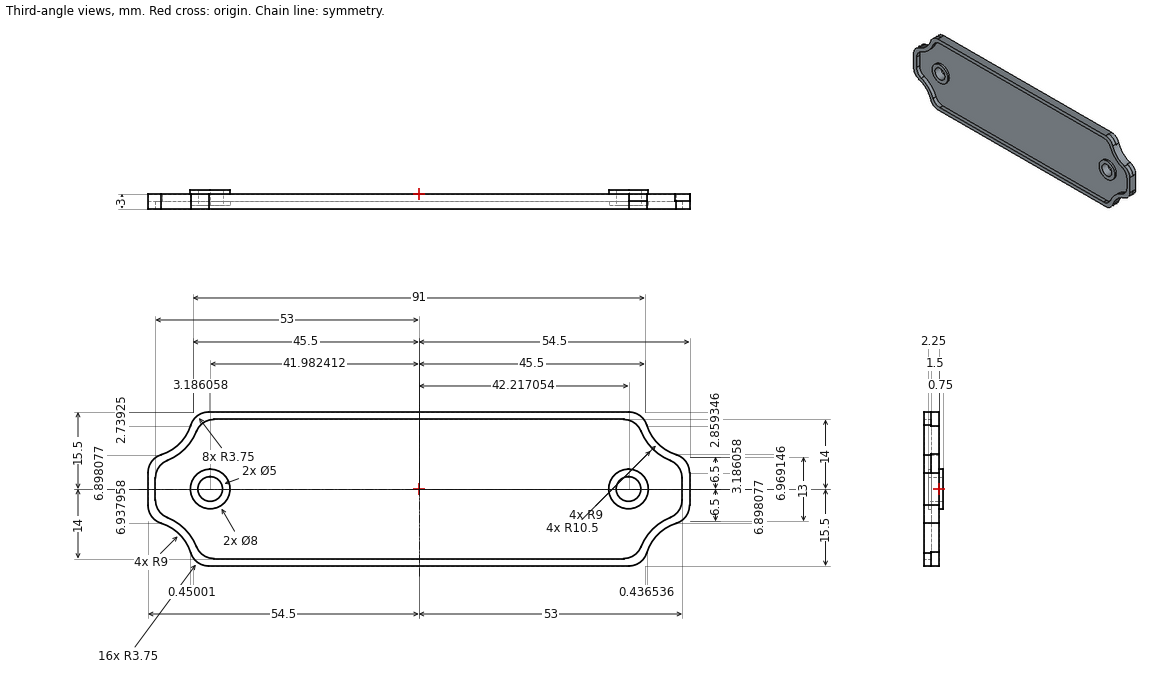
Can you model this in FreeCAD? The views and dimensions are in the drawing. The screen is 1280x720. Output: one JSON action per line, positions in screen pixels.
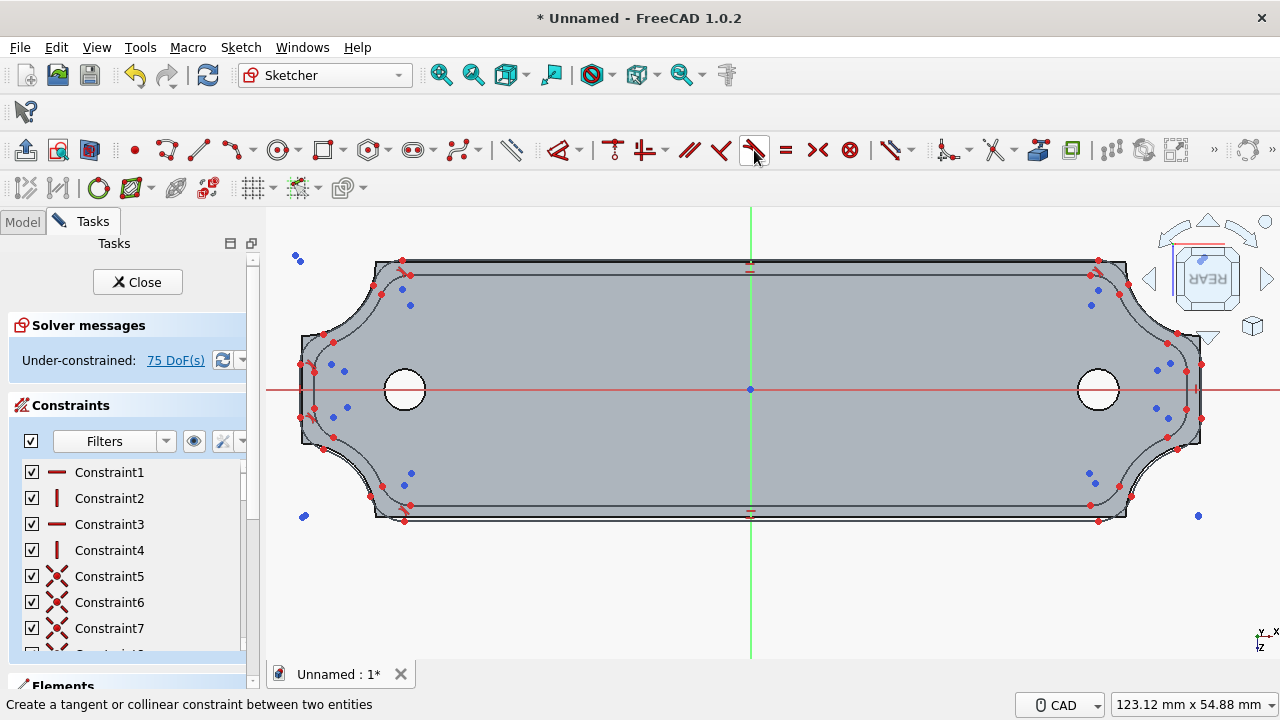
{"action": "left_click", "coordinate": [613, 521]}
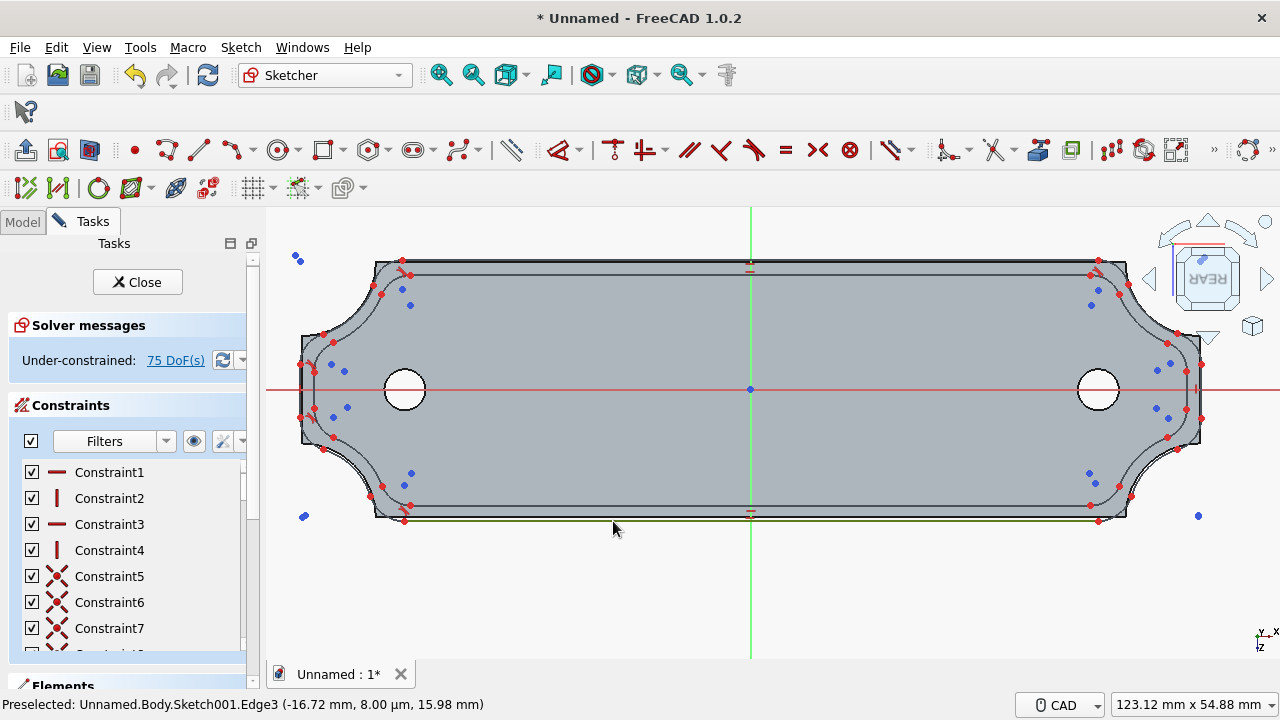
{"action": "left_click", "coordinate": [1111, 518]}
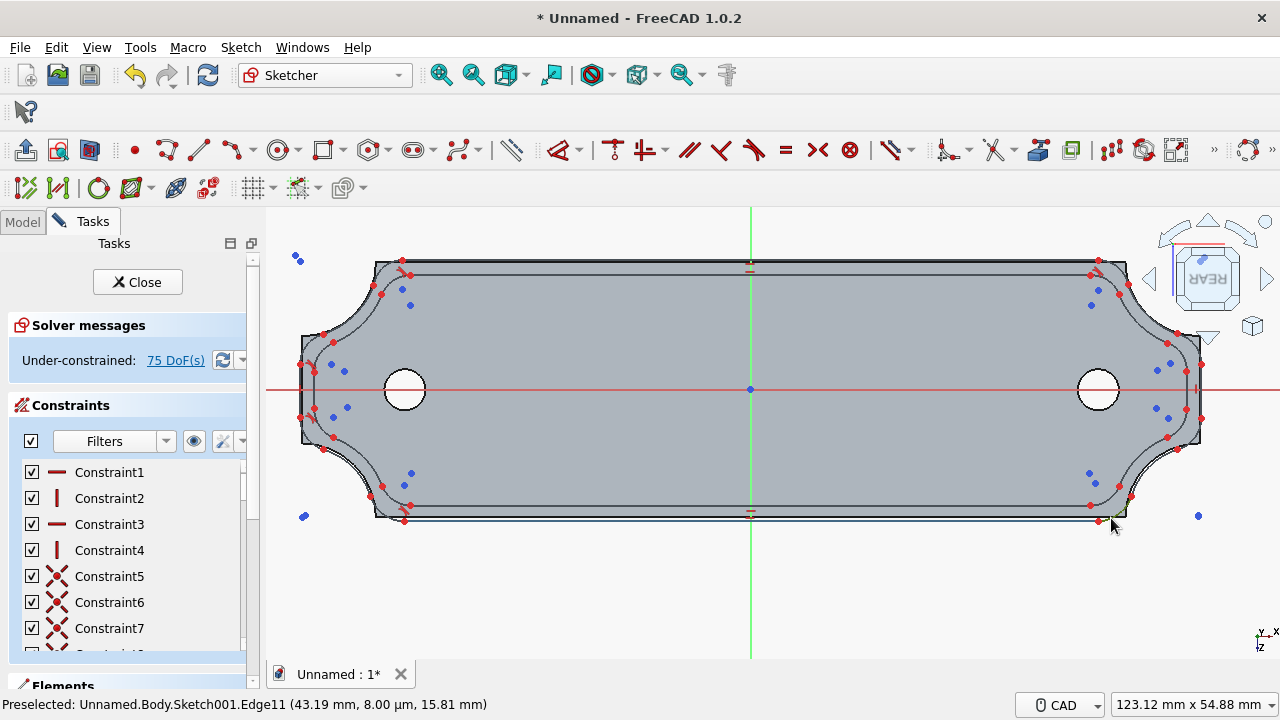
{"action": "left_click", "coordinate": [754, 150]}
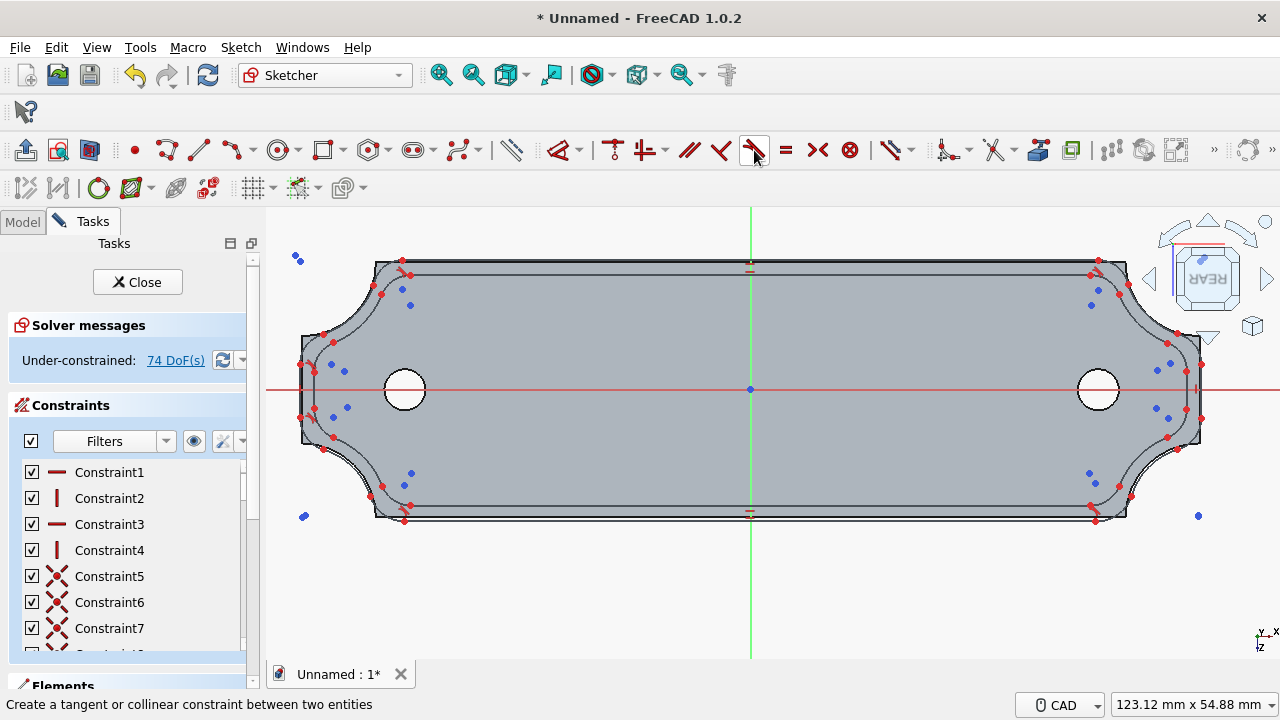
{"action": "scroll", "coordinate": [611, 521], "scroll_direction": "down", "scroll_amount": 2}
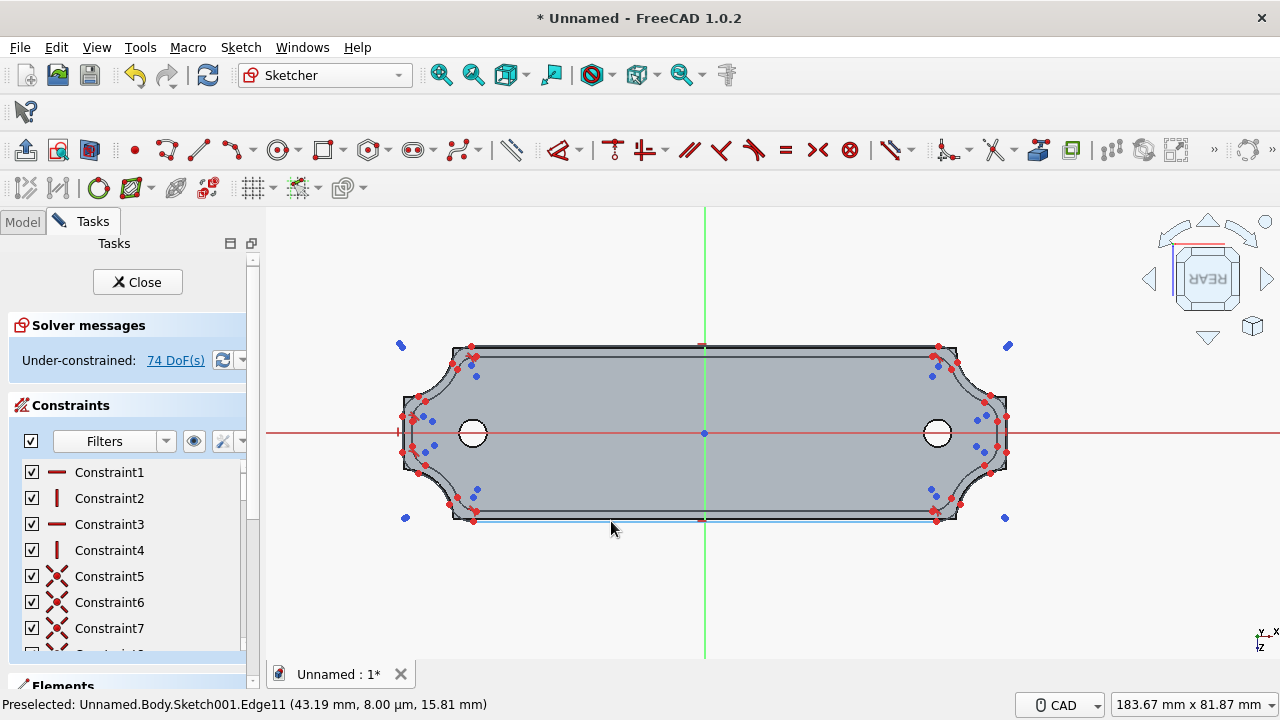
{"action": "scroll", "coordinate": [1007, 442], "scroll_direction": "up", "scroll_amount": 3}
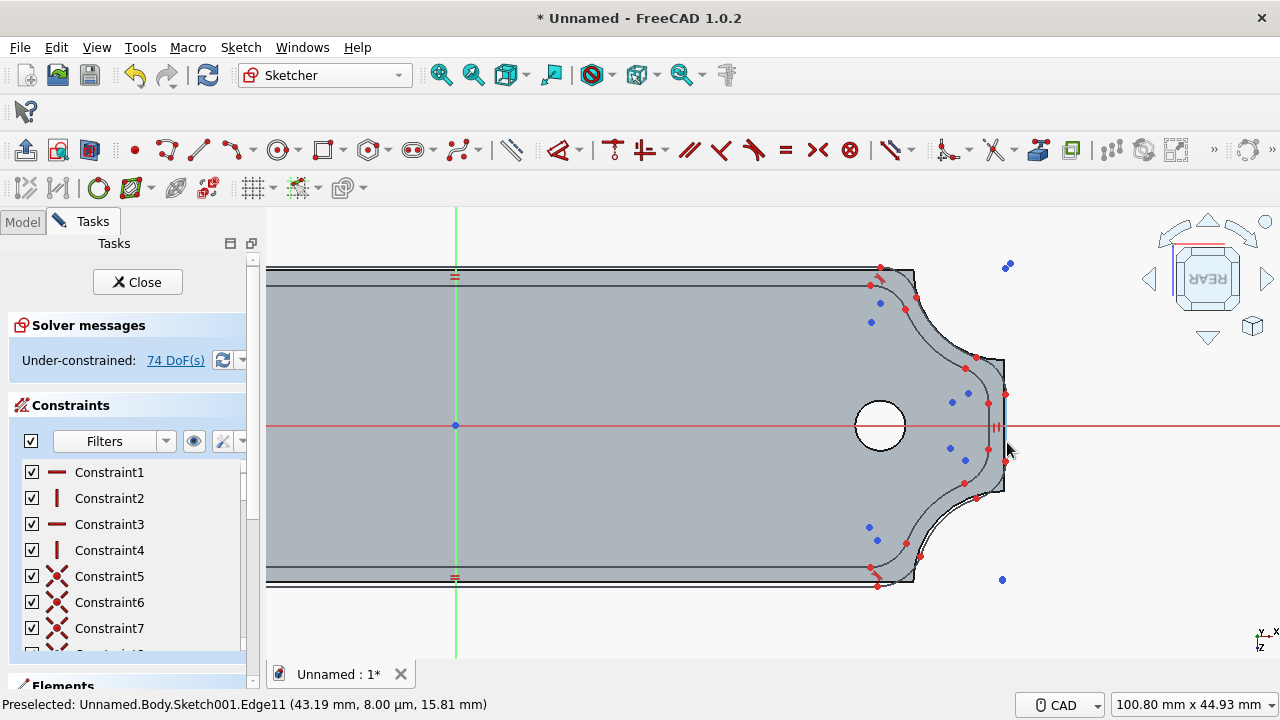
{"action": "left_click", "coordinate": [1006, 441]}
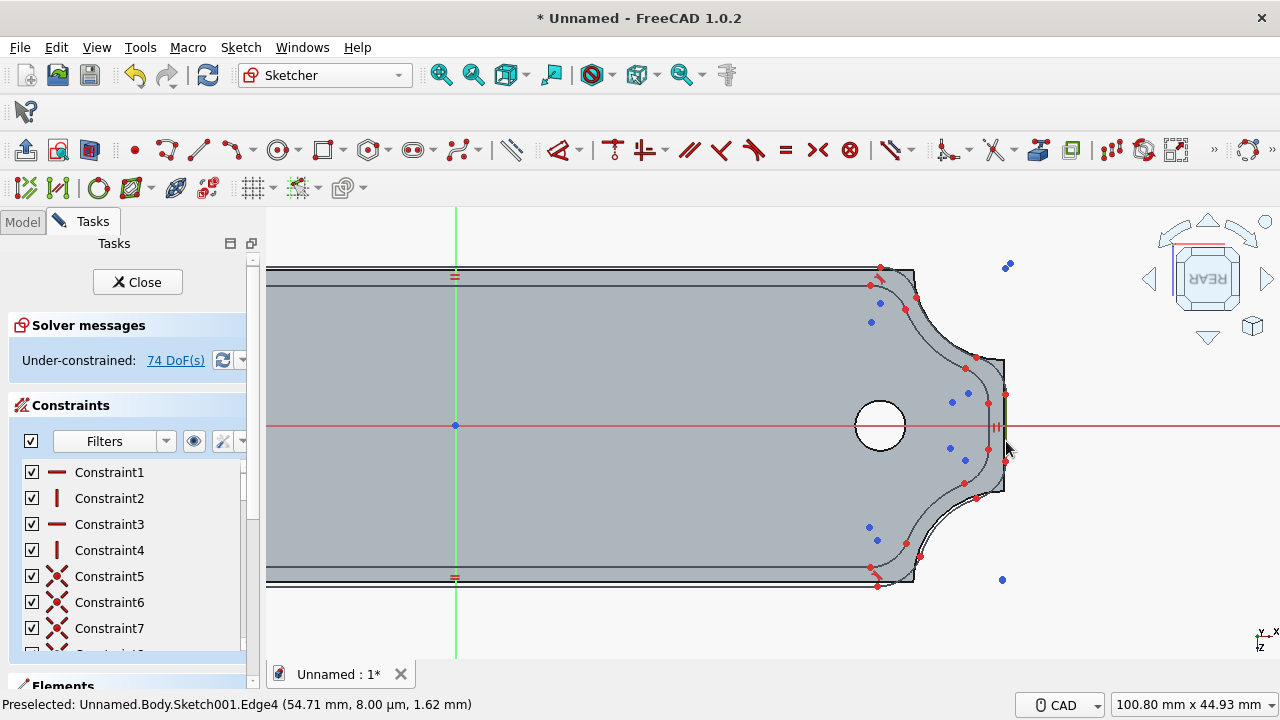
{"action": "left_click", "coordinate": [990, 492]}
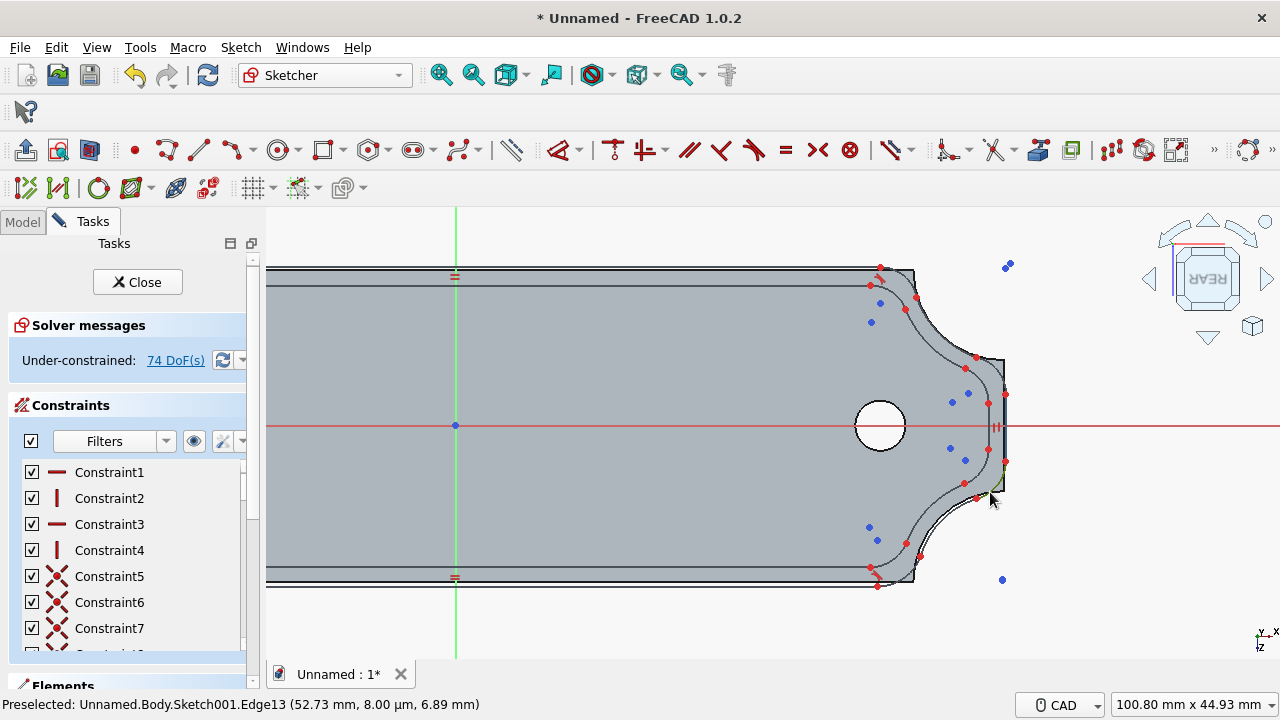
{"action": "left_click", "coordinate": [754, 150]}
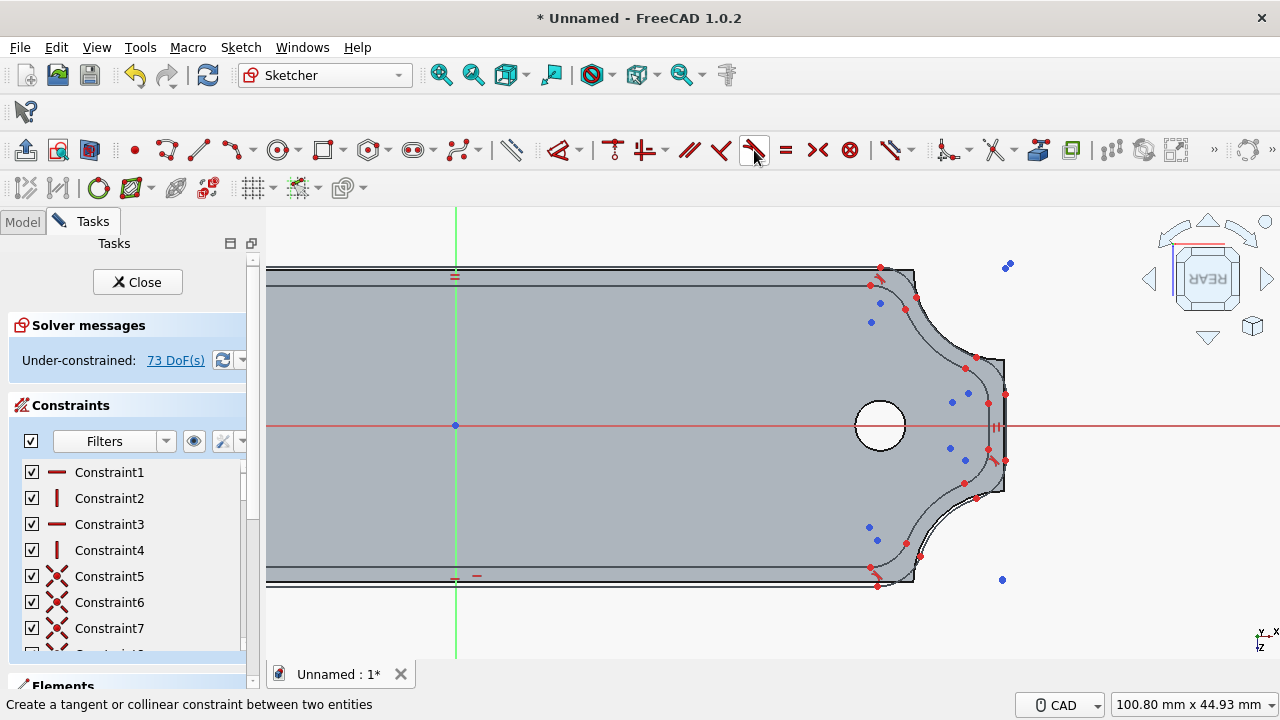
{"action": "left_click", "coordinate": [1006, 441]}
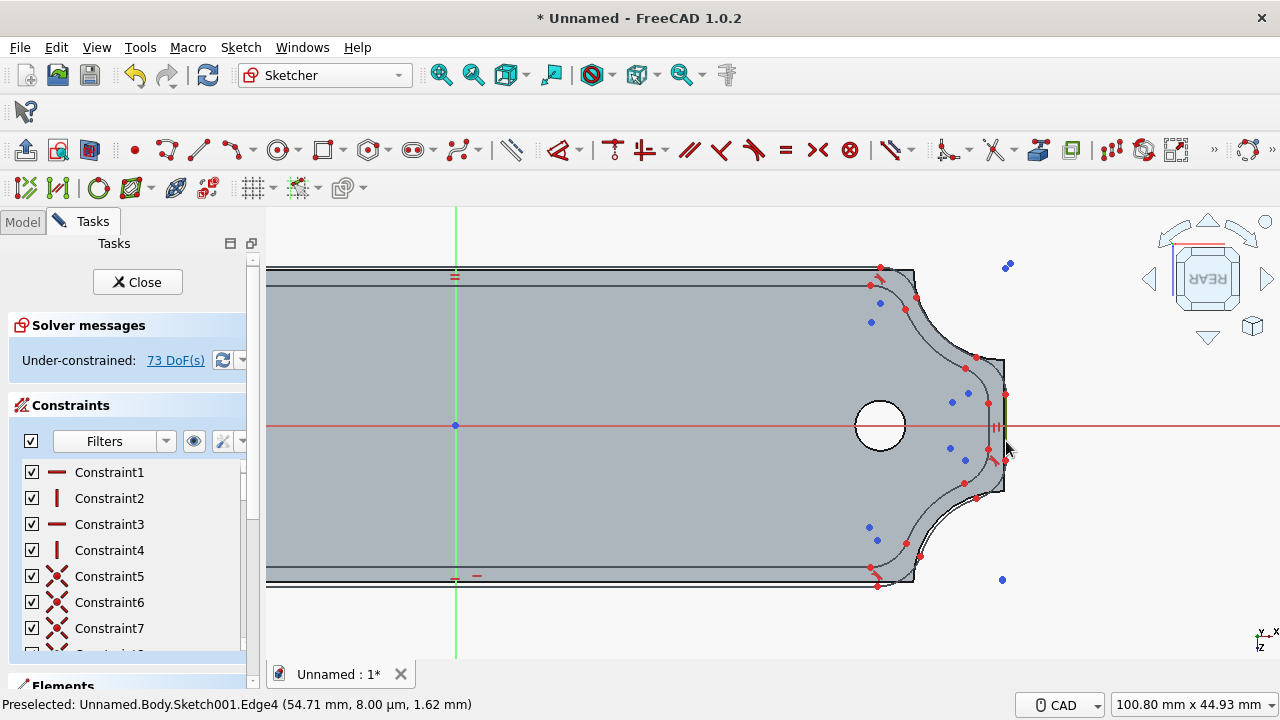
{"action": "left_click", "coordinate": [1003, 380]}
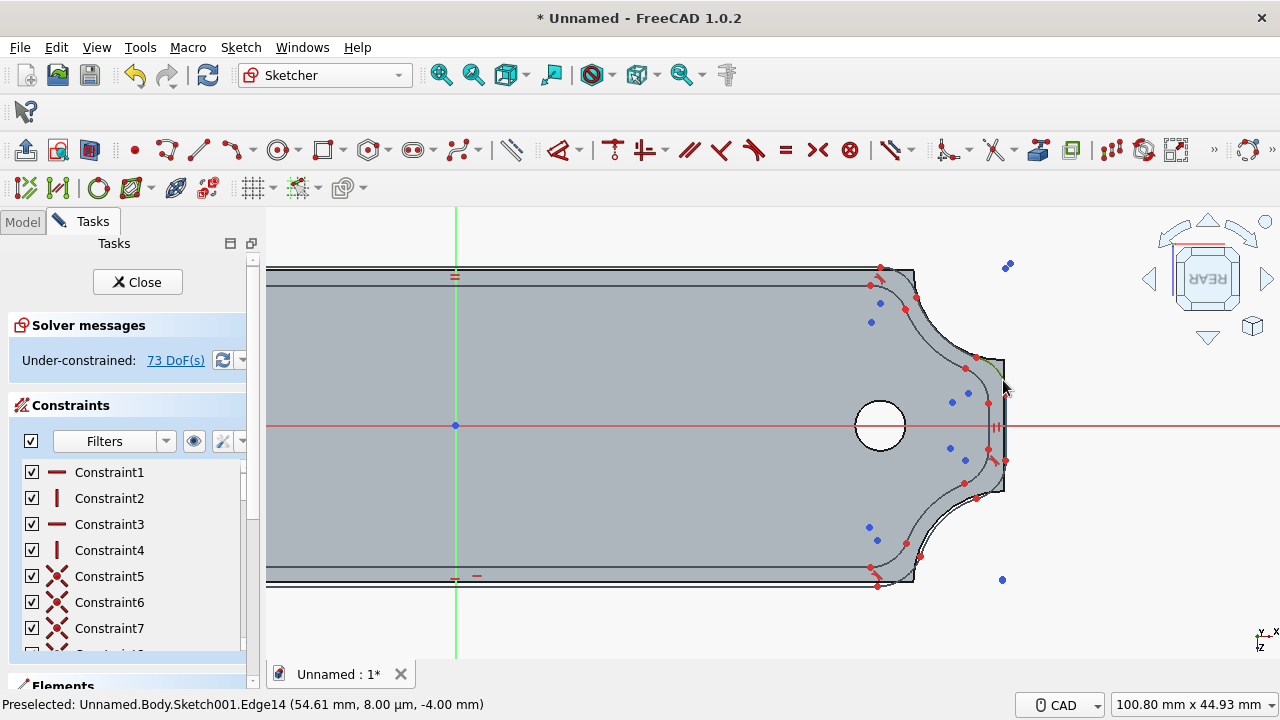
{"action": "left_click", "coordinate": [754, 150]}